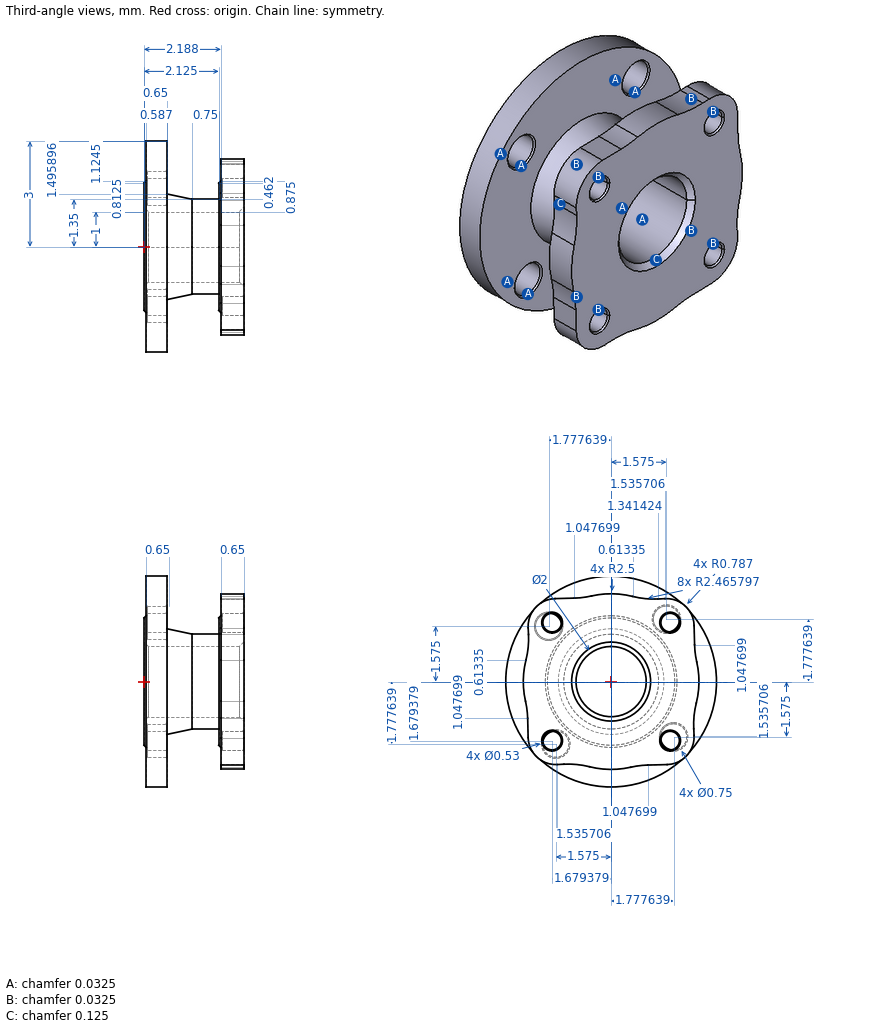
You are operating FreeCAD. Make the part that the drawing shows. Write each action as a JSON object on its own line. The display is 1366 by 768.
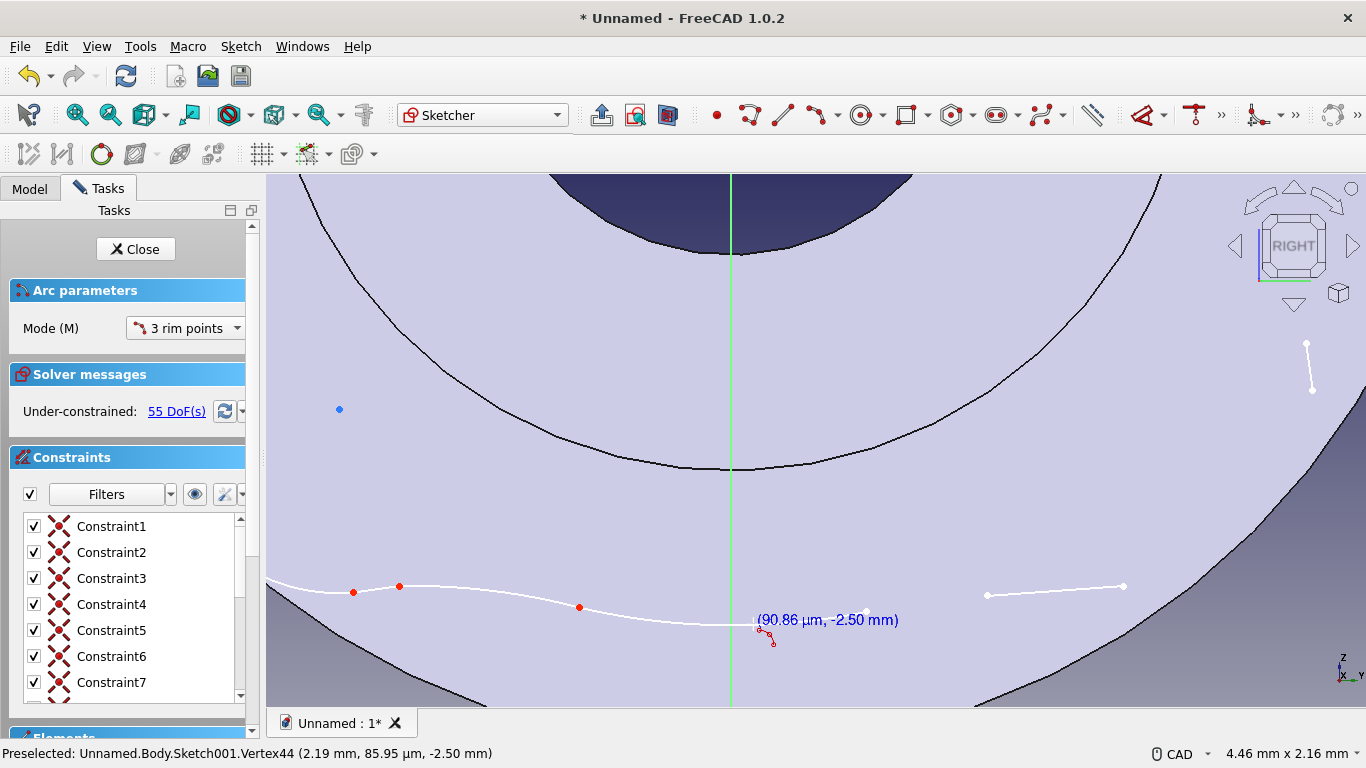
{"action": "scroll", "coordinate": [755, 627], "scroll_direction": "down", "scroll_amount": 6}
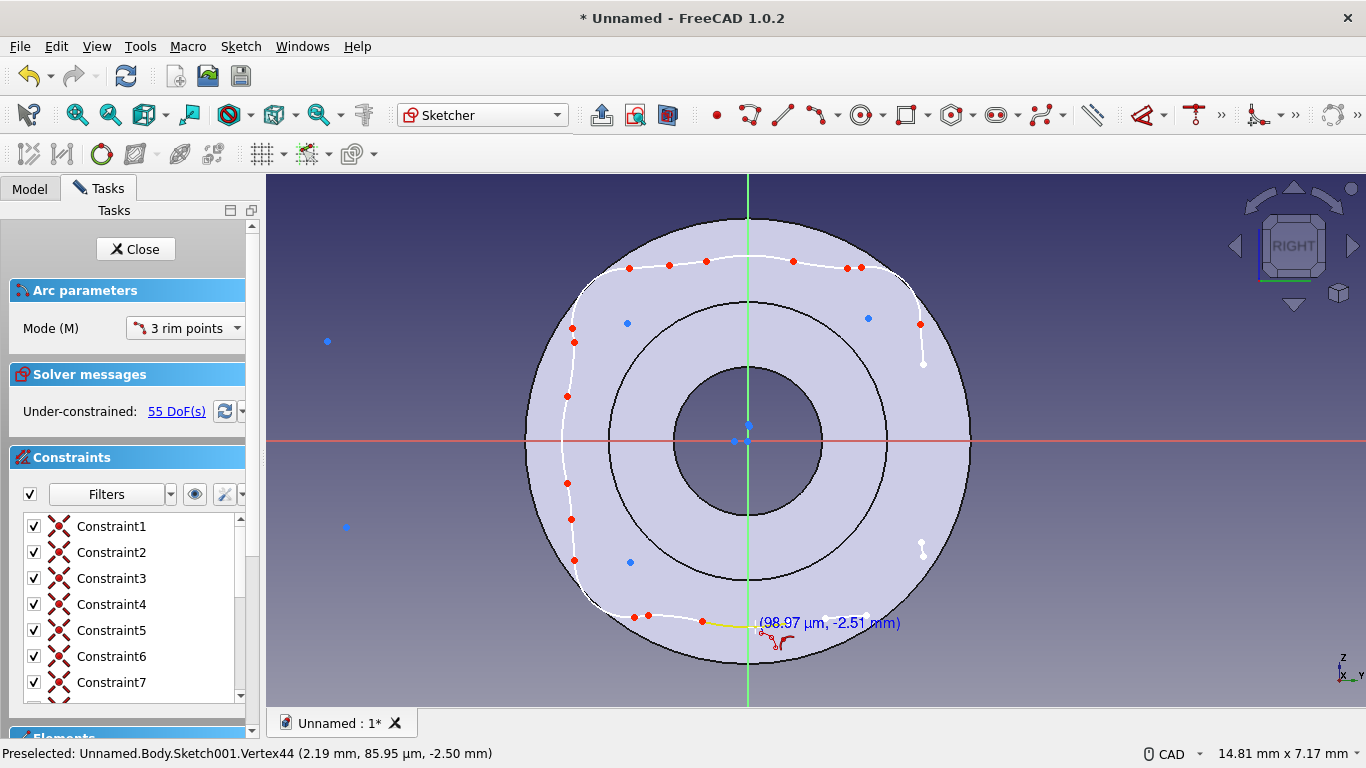
{"action": "left_click", "coordinate": [789, 623]}
{"action": "left_click", "coordinate": [825, 618]}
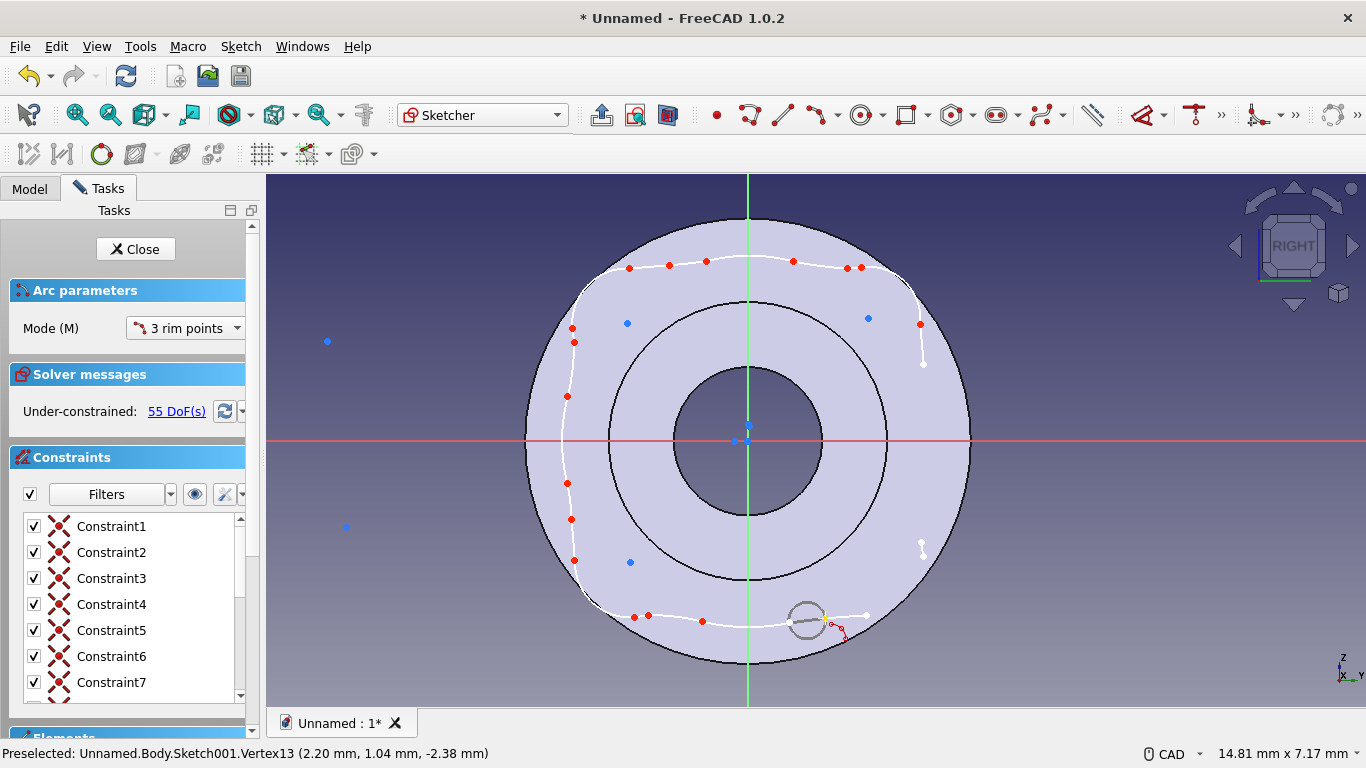
{"action": "scroll", "coordinate": [808, 619], "scroll_direction": "up", "scroll_amount": 15}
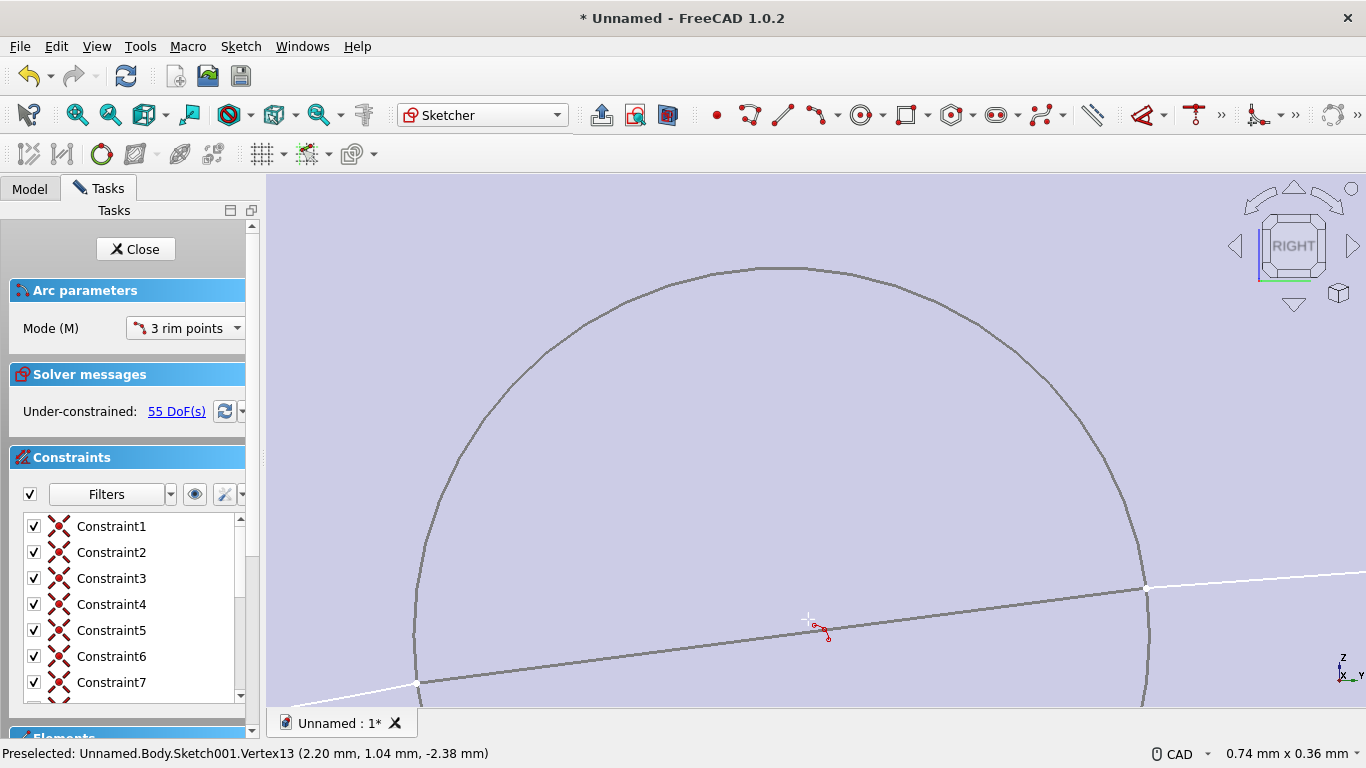
{"action": "left_click", "coordinate": [789, 604]}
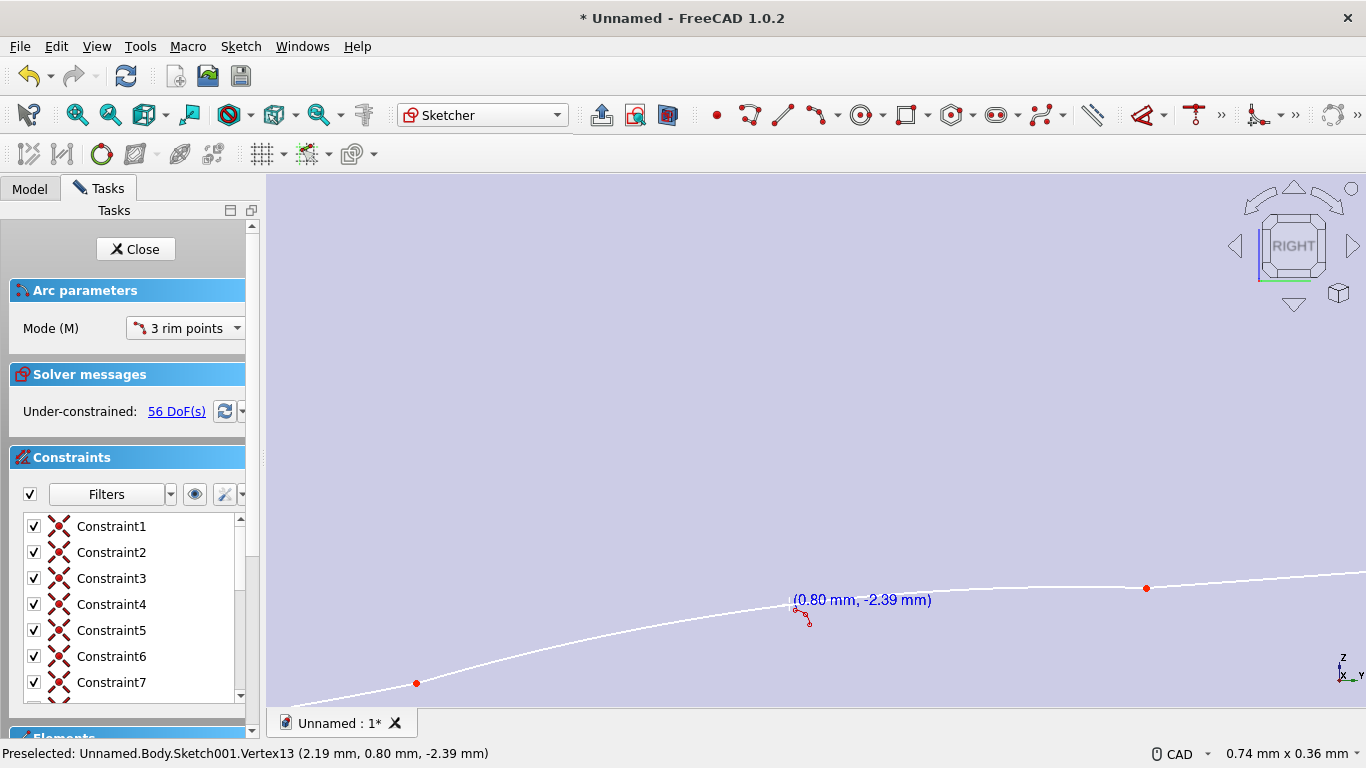
{"action": "scroll", "coordinate": [808, 619], "scroll_direction": "down", "scroll_amount": 15}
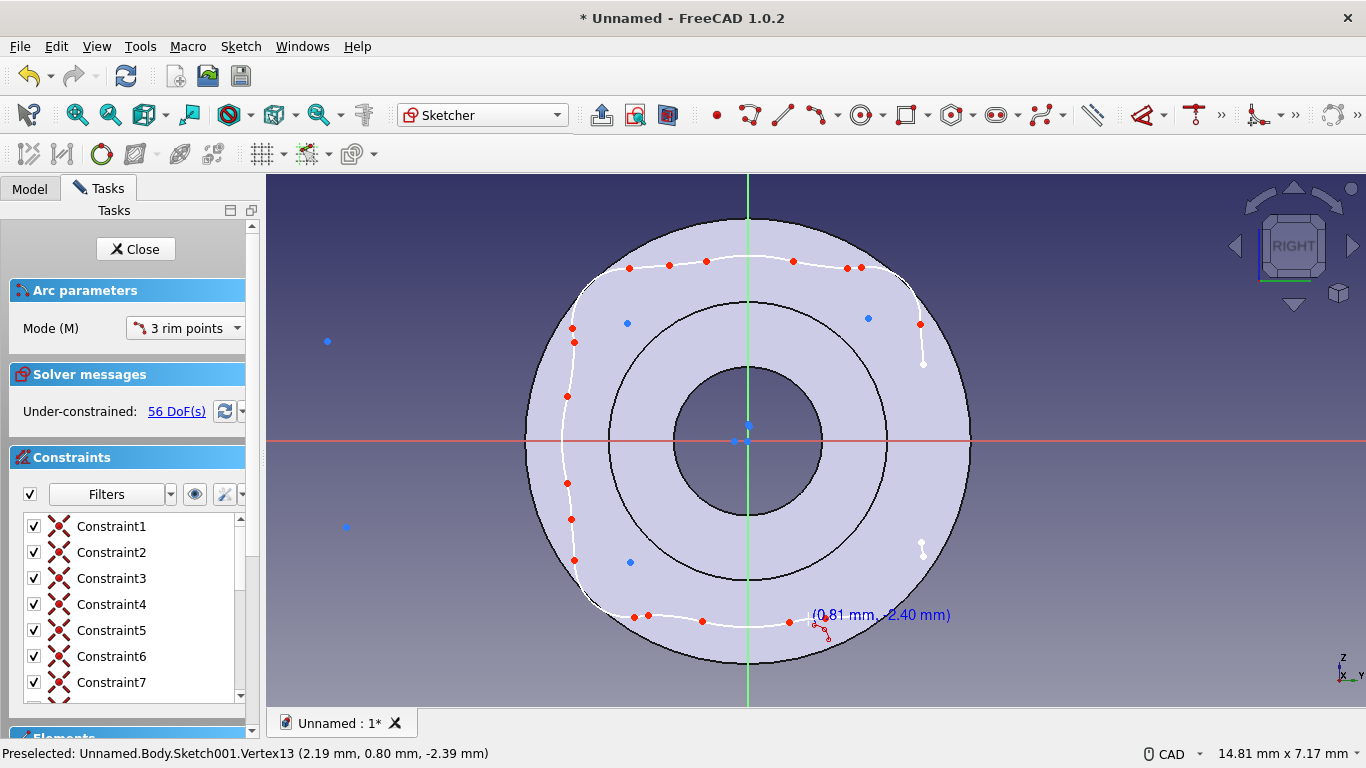
{"action": "left_click", "coordinate": [866, 615]}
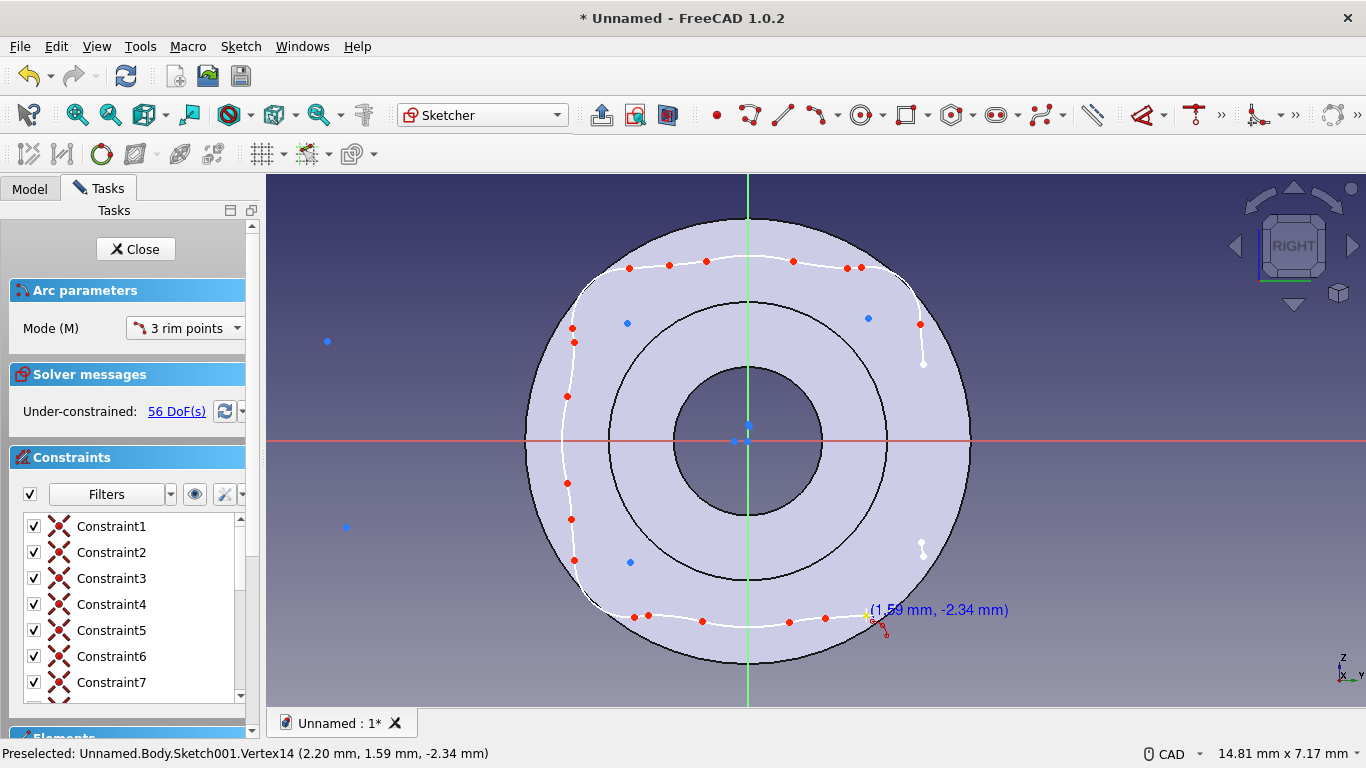
{"action": "scroll", "coordinate": [923, 555], "scroll_direction": "up", "scroll_amount": 4}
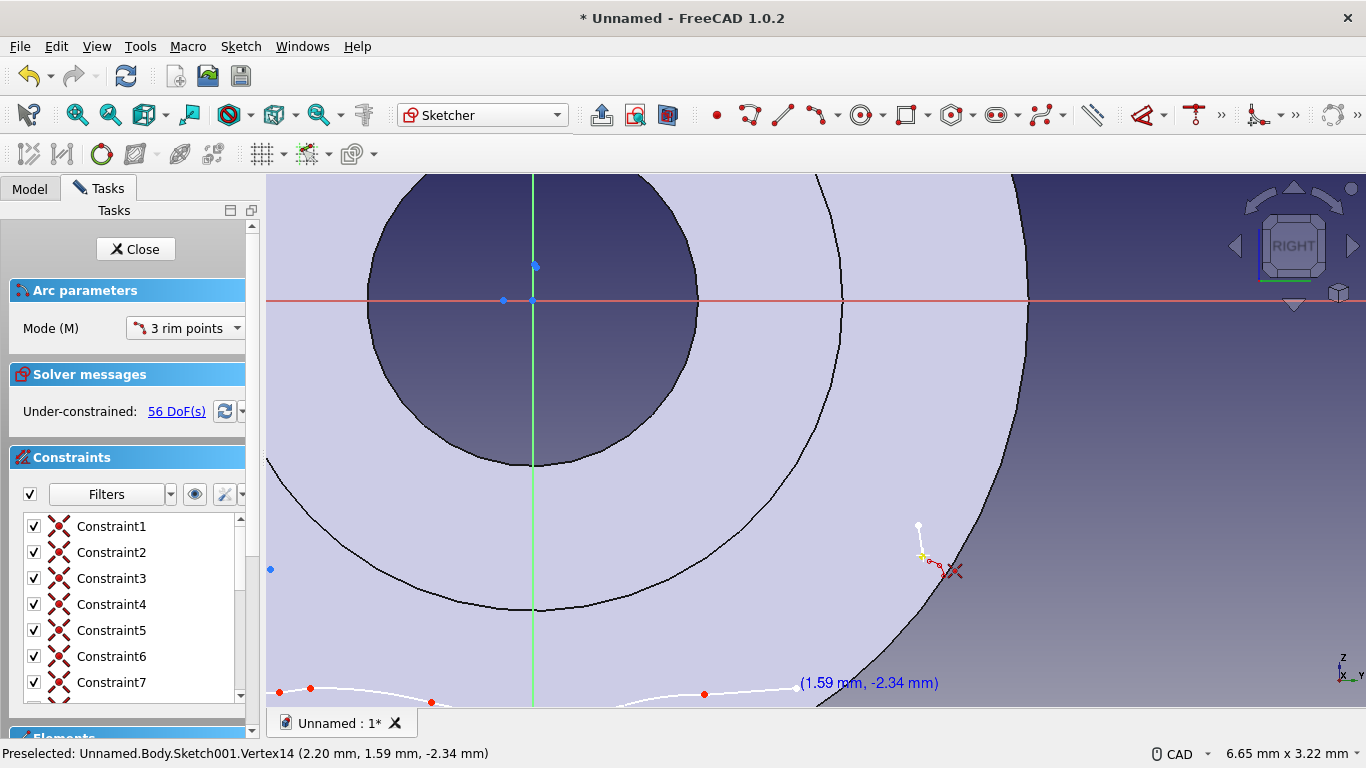
{"action": "left_click", "coordinate": [923, 557]}
{"action": "left_click", "coordinate": [889, 650]}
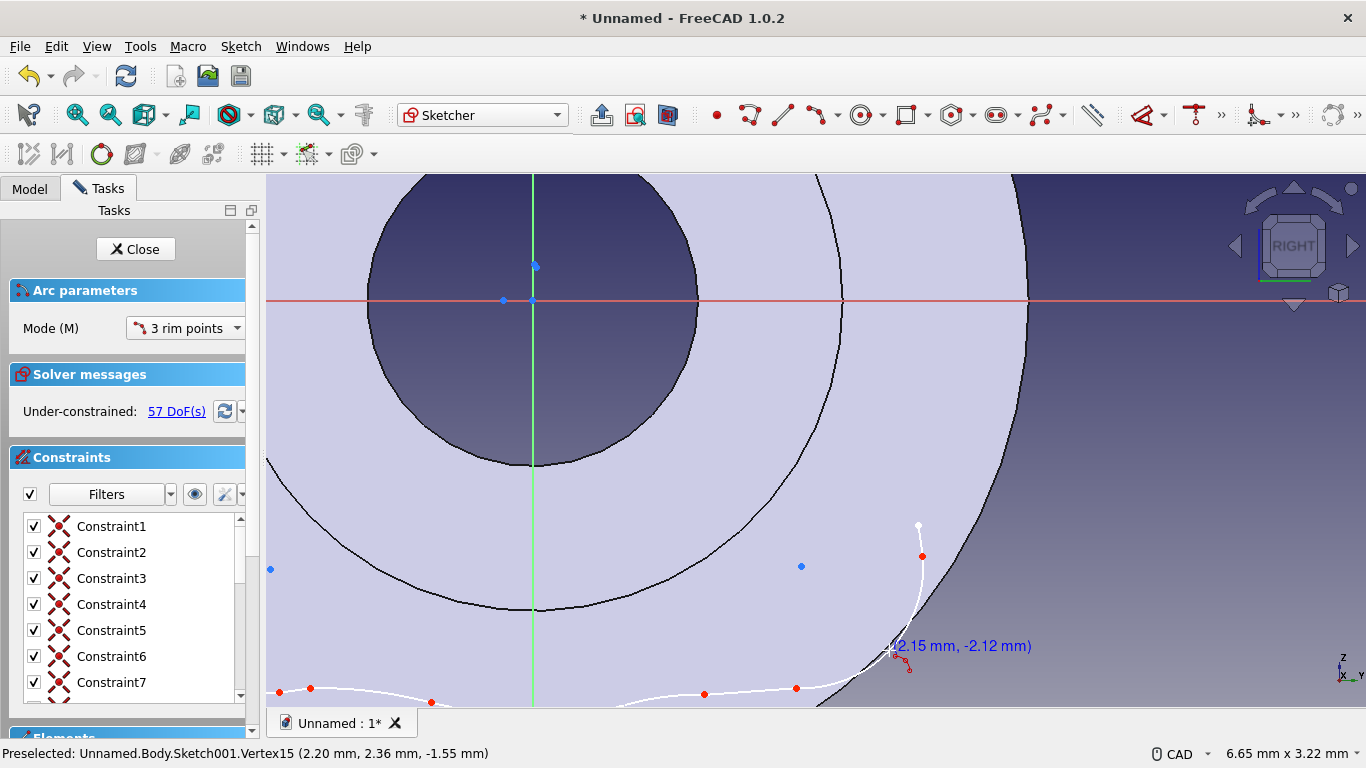
{"action": "left_click", "coordinate": [919, 526]}
{"action": "left_click", "coordinate": [933, 402]}